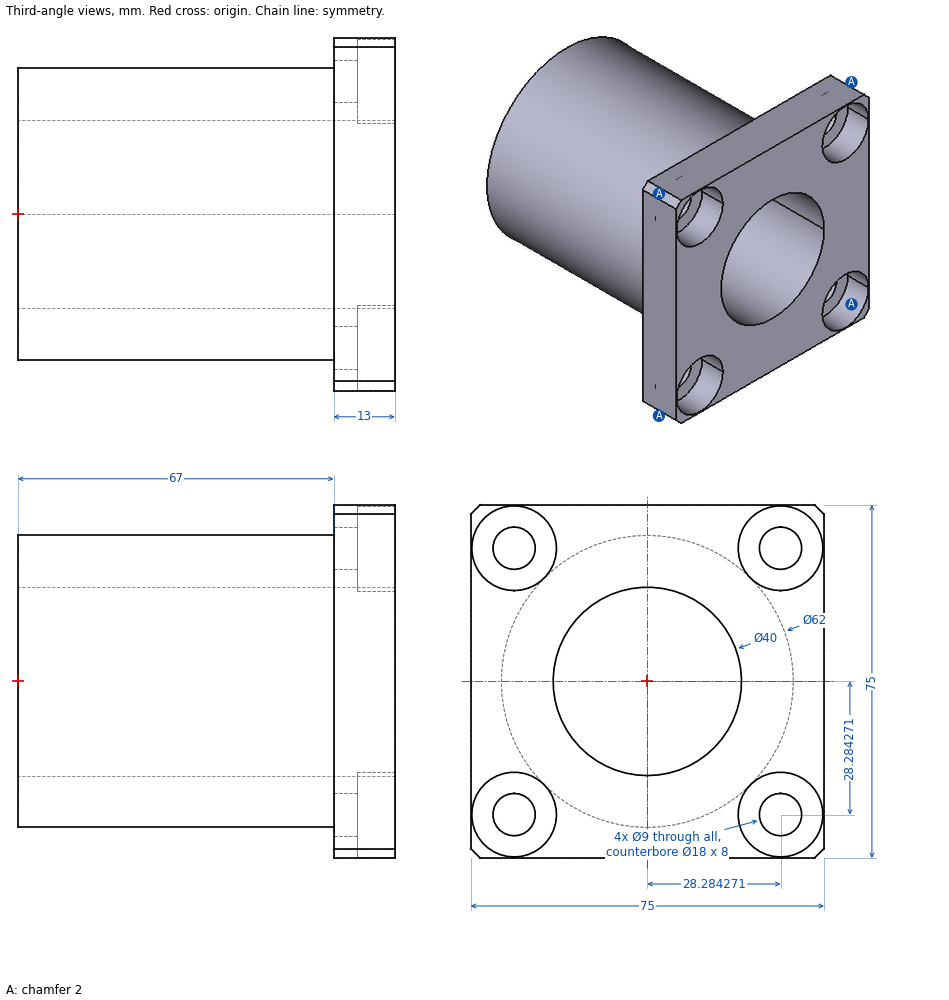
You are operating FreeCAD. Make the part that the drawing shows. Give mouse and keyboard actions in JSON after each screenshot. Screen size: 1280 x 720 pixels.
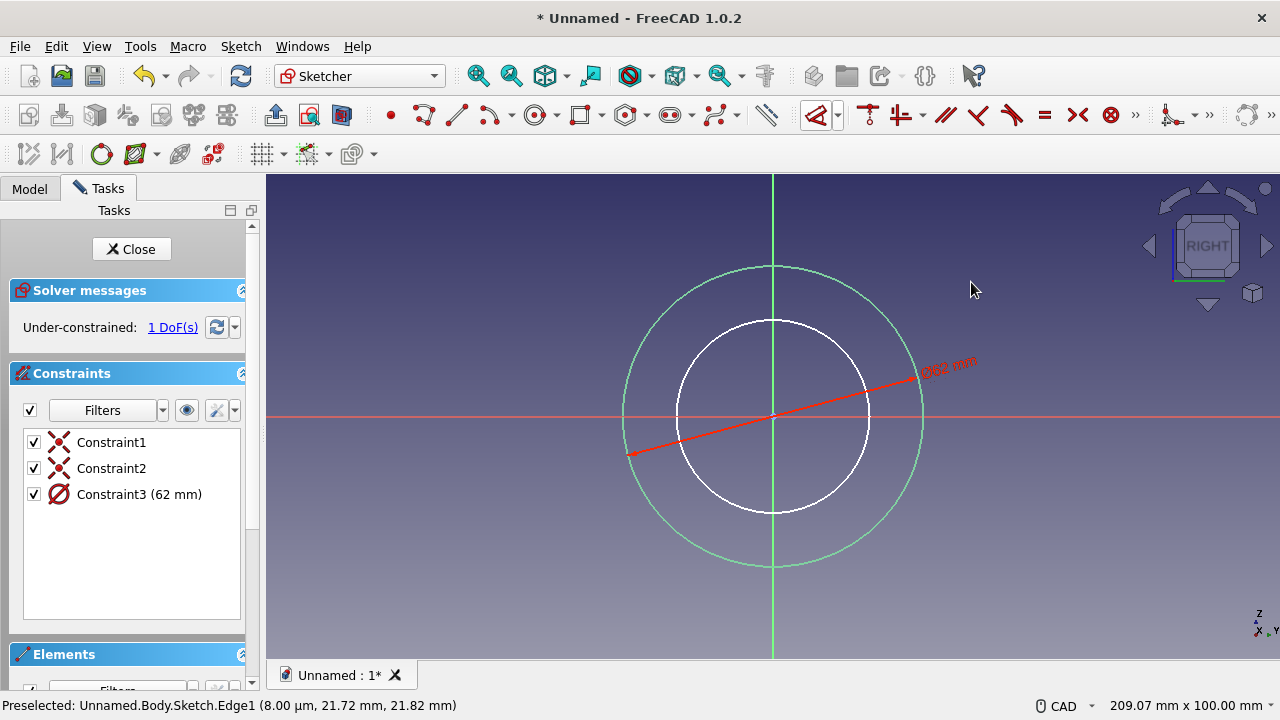
{"action": "left_click", "coordinate": [841, 348]}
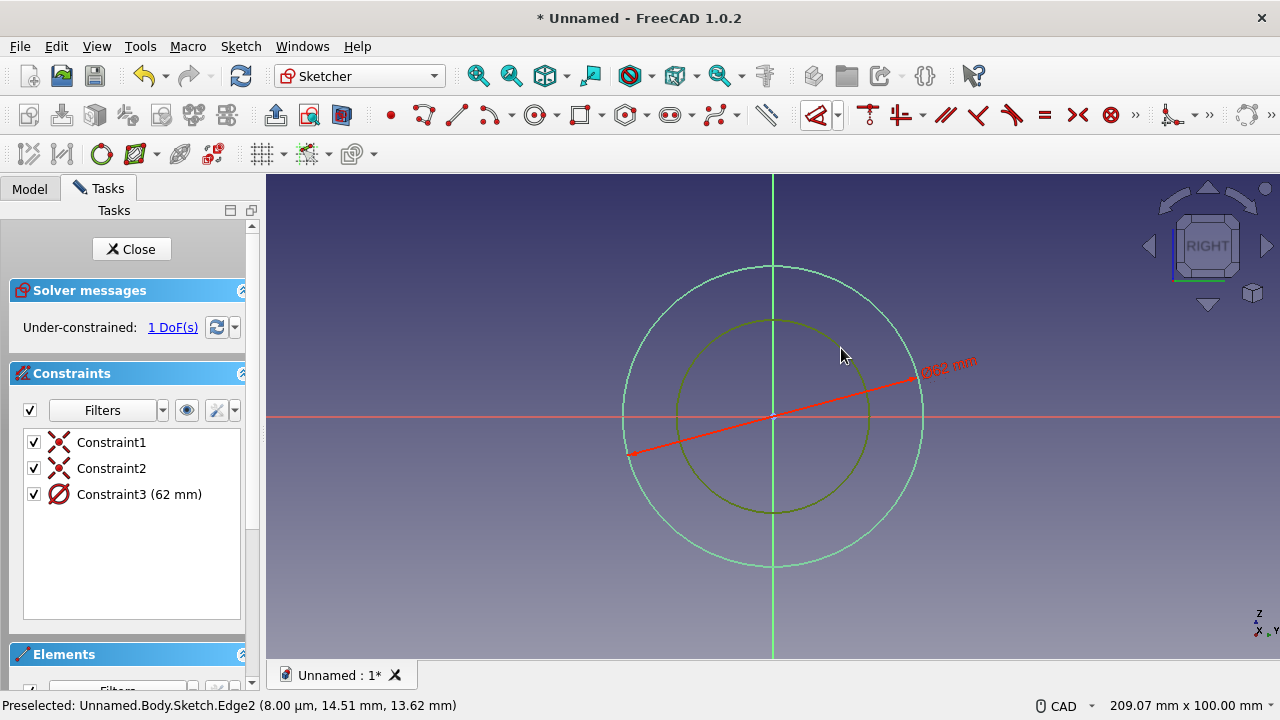
{"action": "key", "text": "k o"}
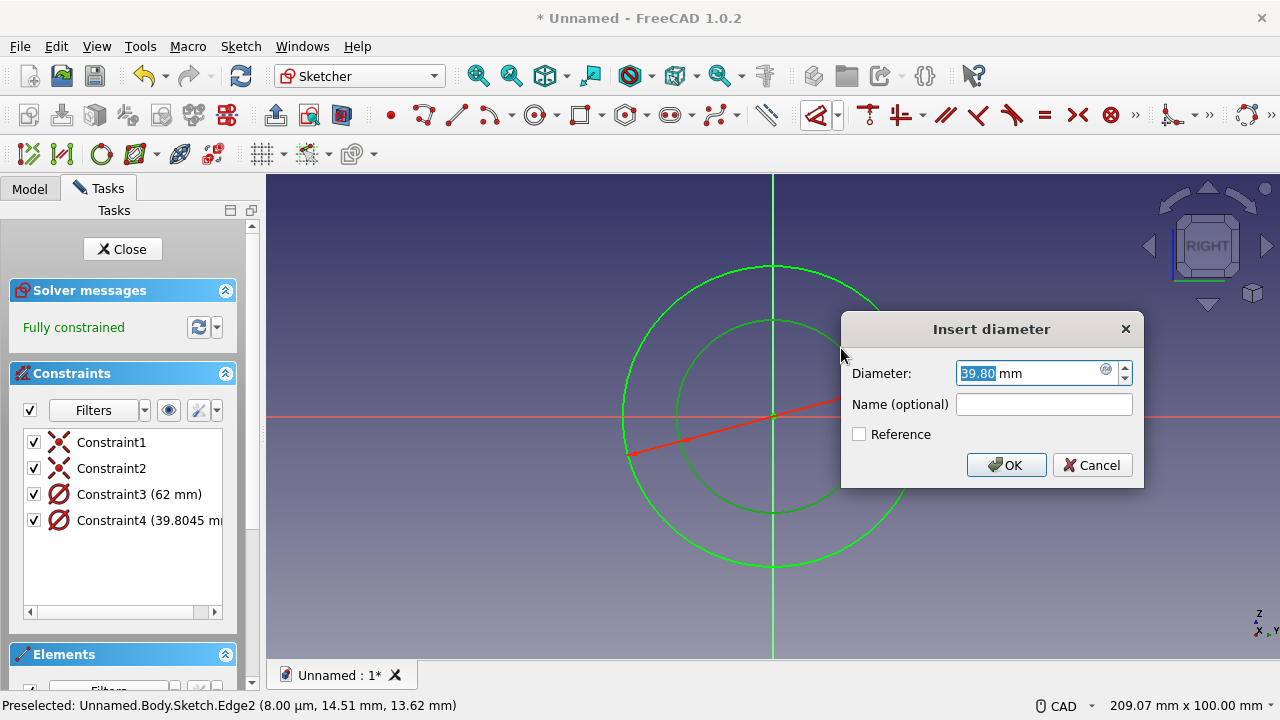
{"action": "type", "text": "40"}
{"action": "key", "text": "Return"}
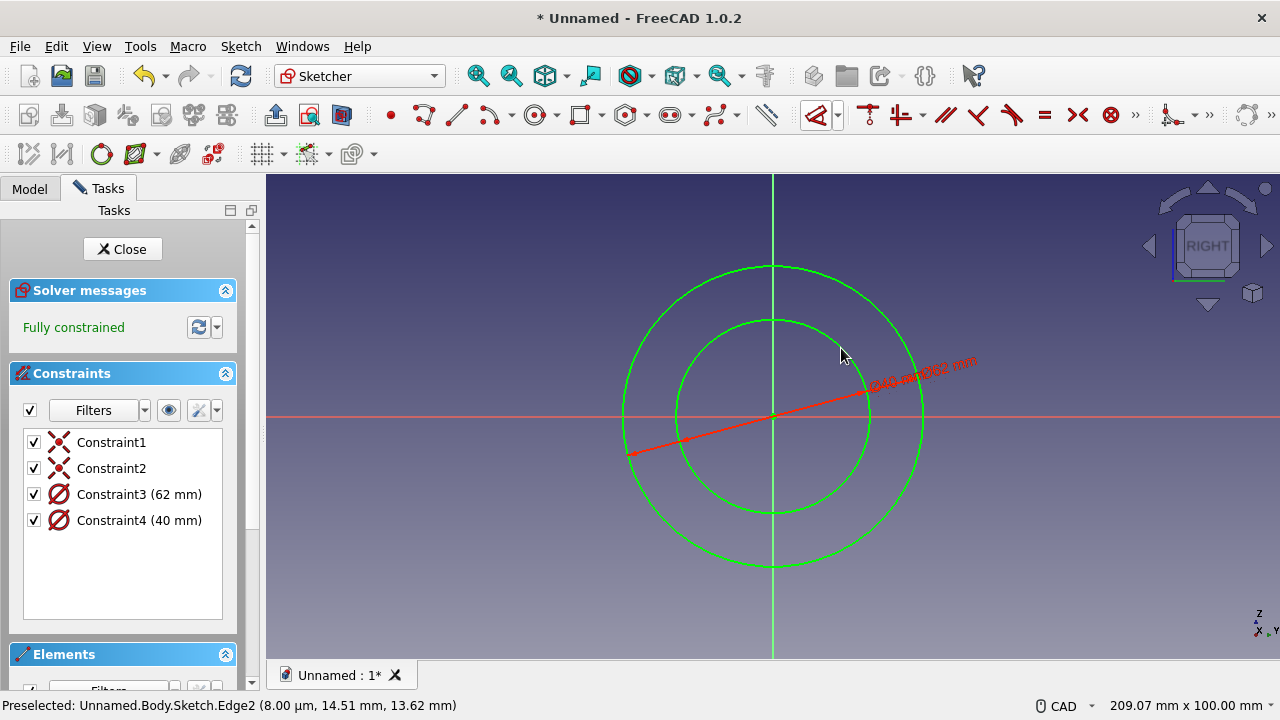
{"action": "left_click", "coordinate": [123, 249]}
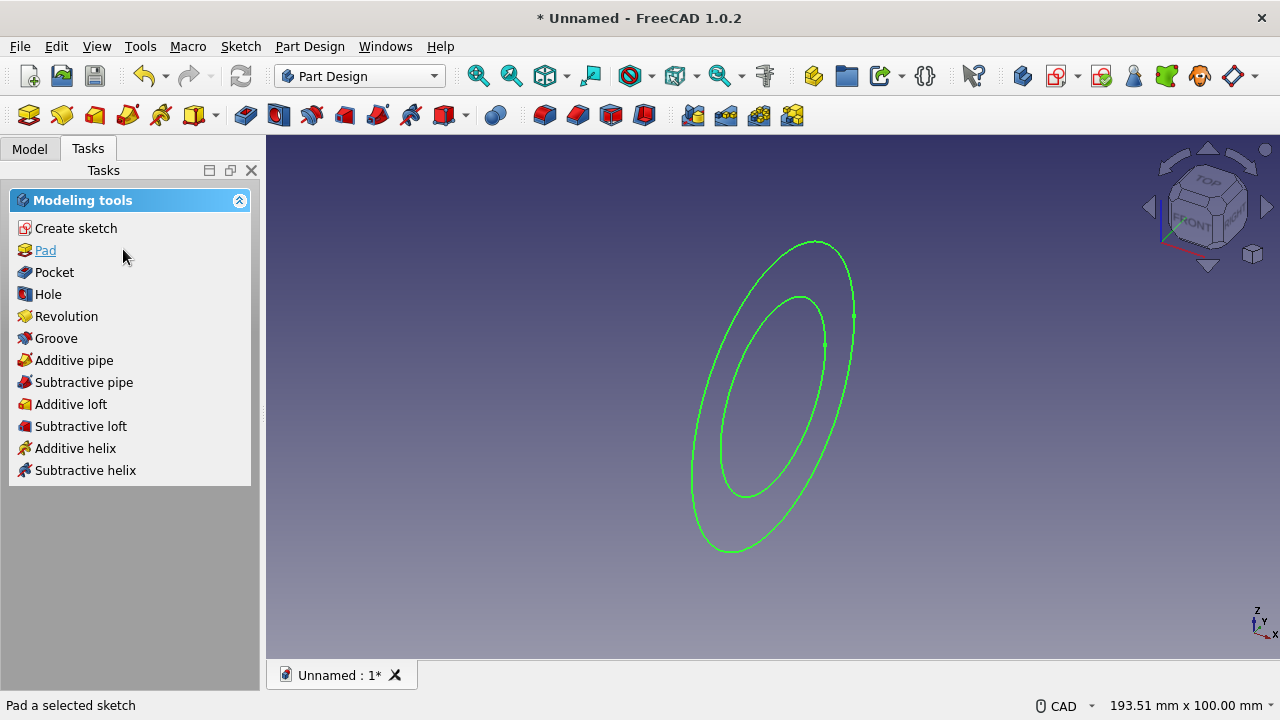
{"action": "left_click", "coordinate": [29, 116]}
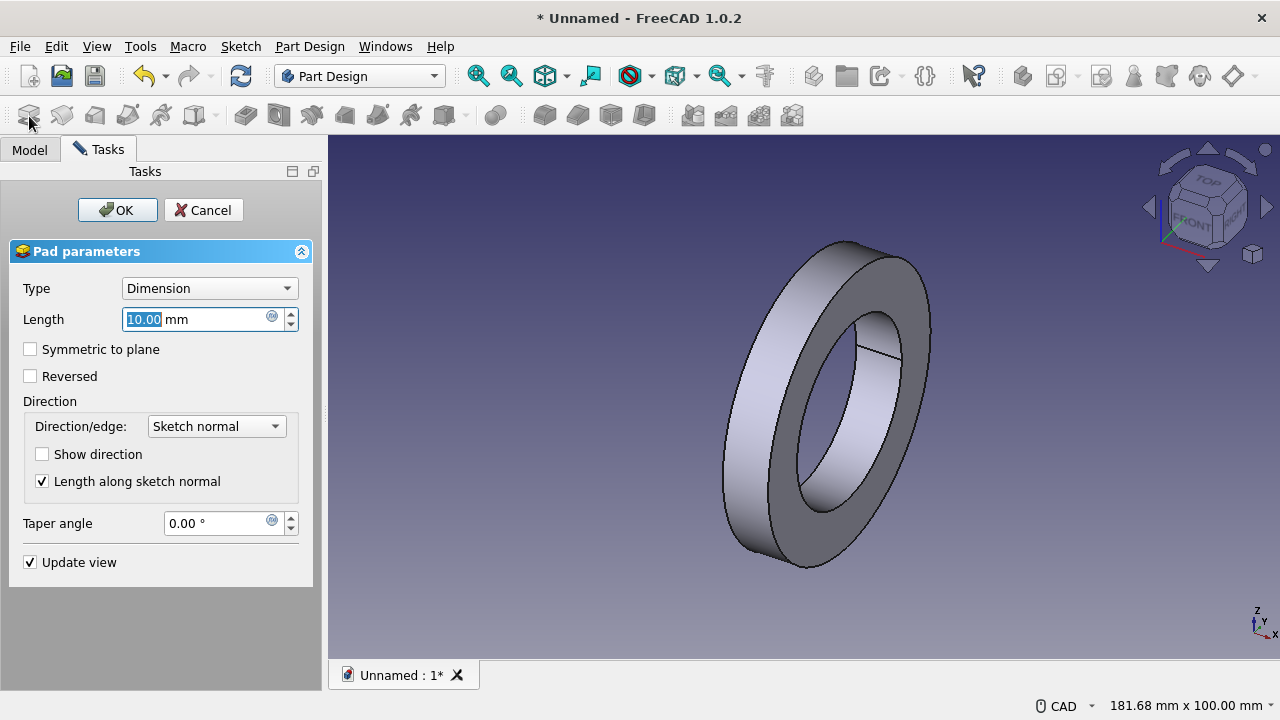
{"action": "type", "text": "67"}
{"action": "key", "text": "Tab"}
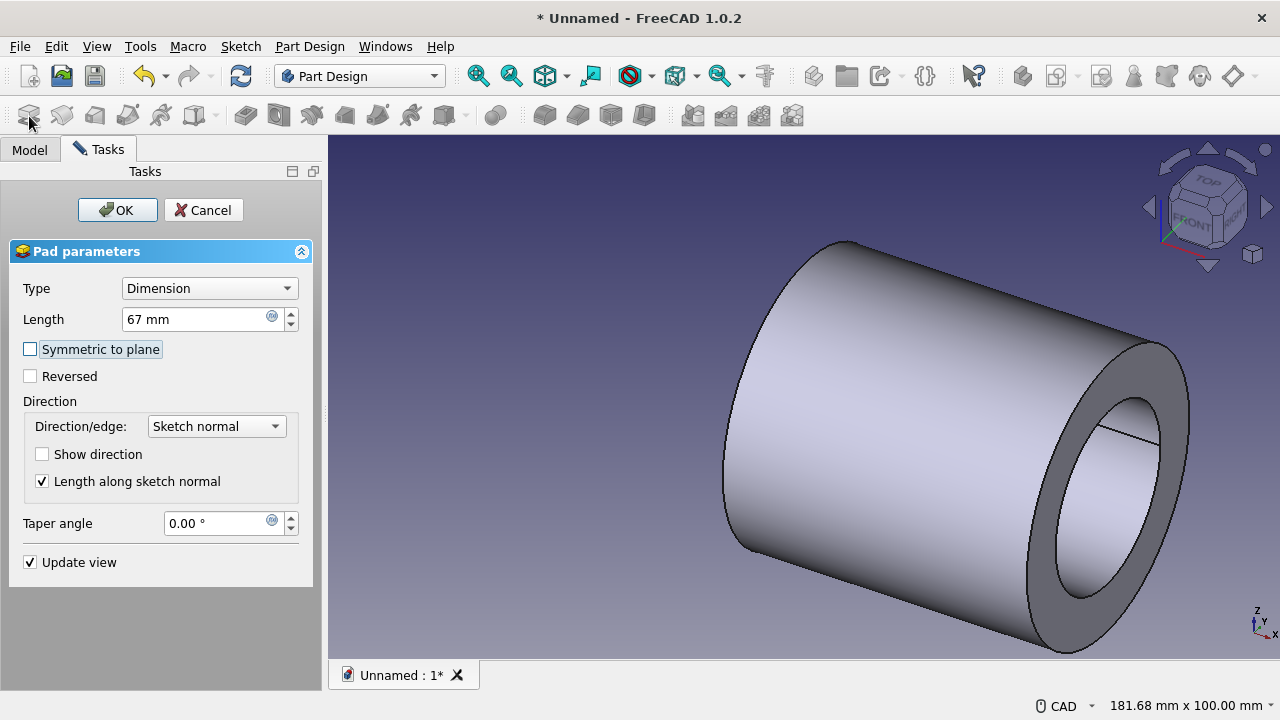
{"action": "left_click", "coordinate": [118, 210]}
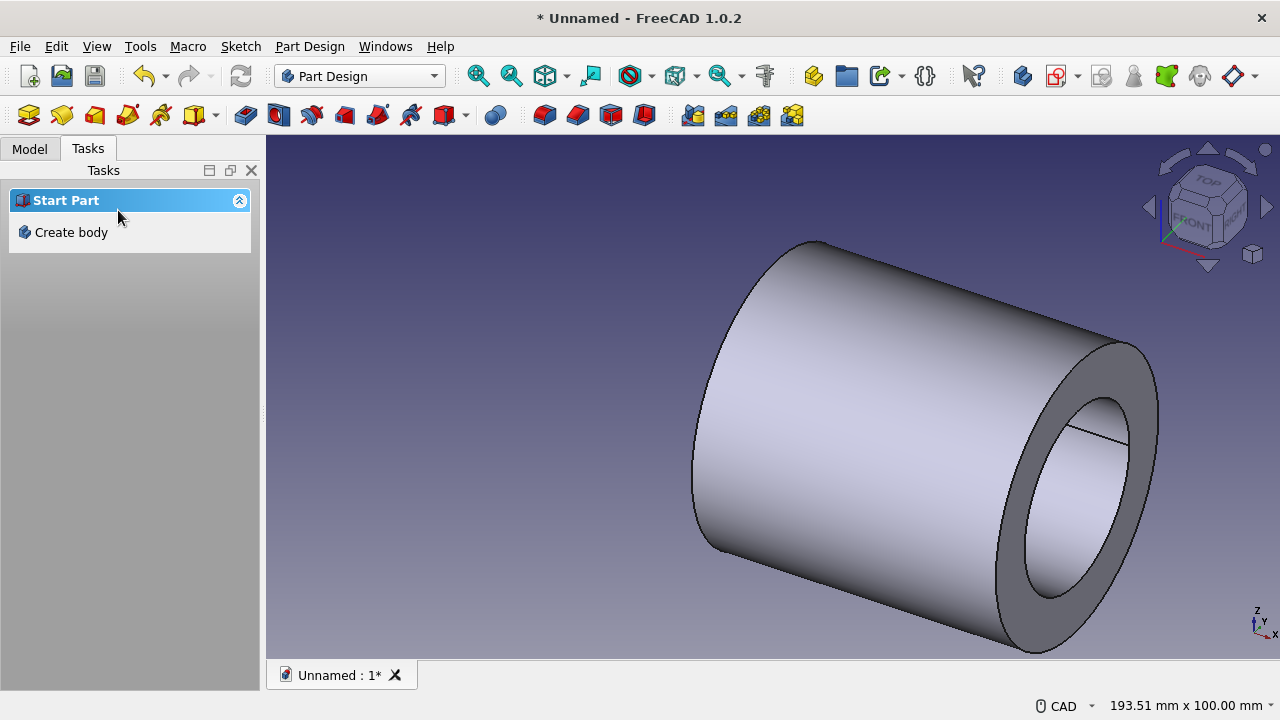
{"action": "left_click", "coordinate": [479, 76]}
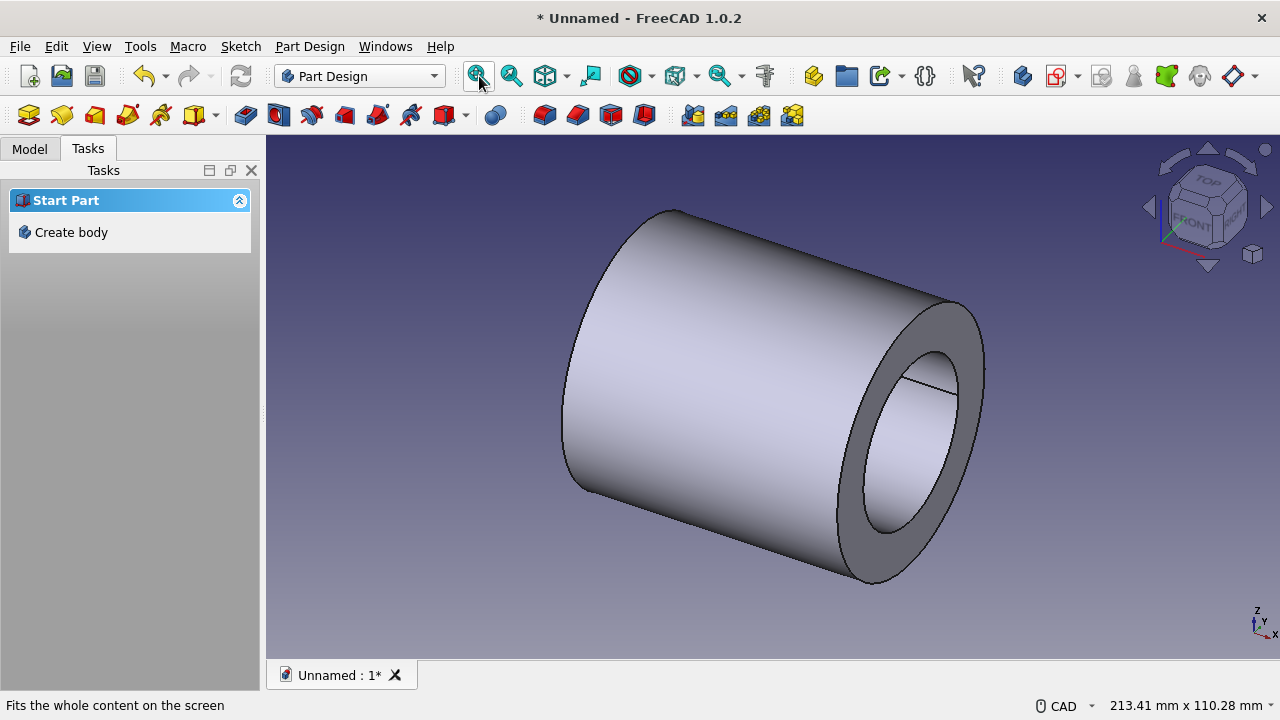
{"action": "left_click", "coordinate": [953, 331]}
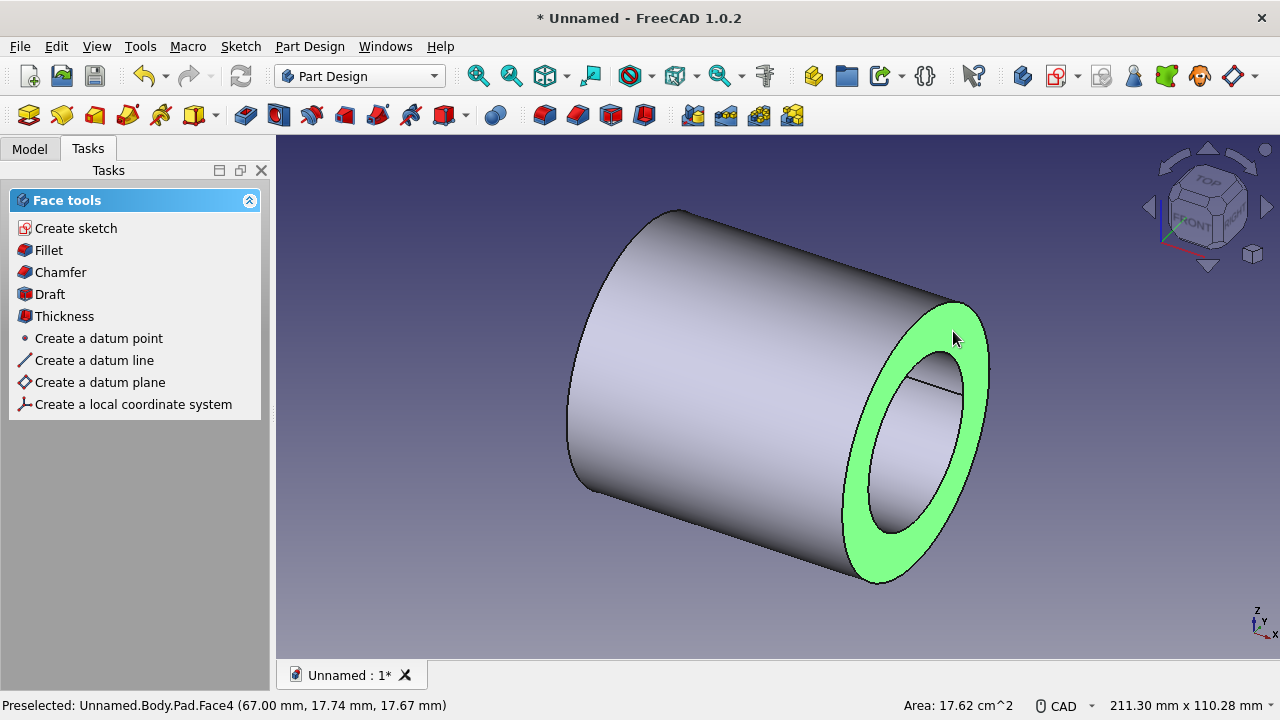
{"action": "left_click", "coordinate": [1056, 76]}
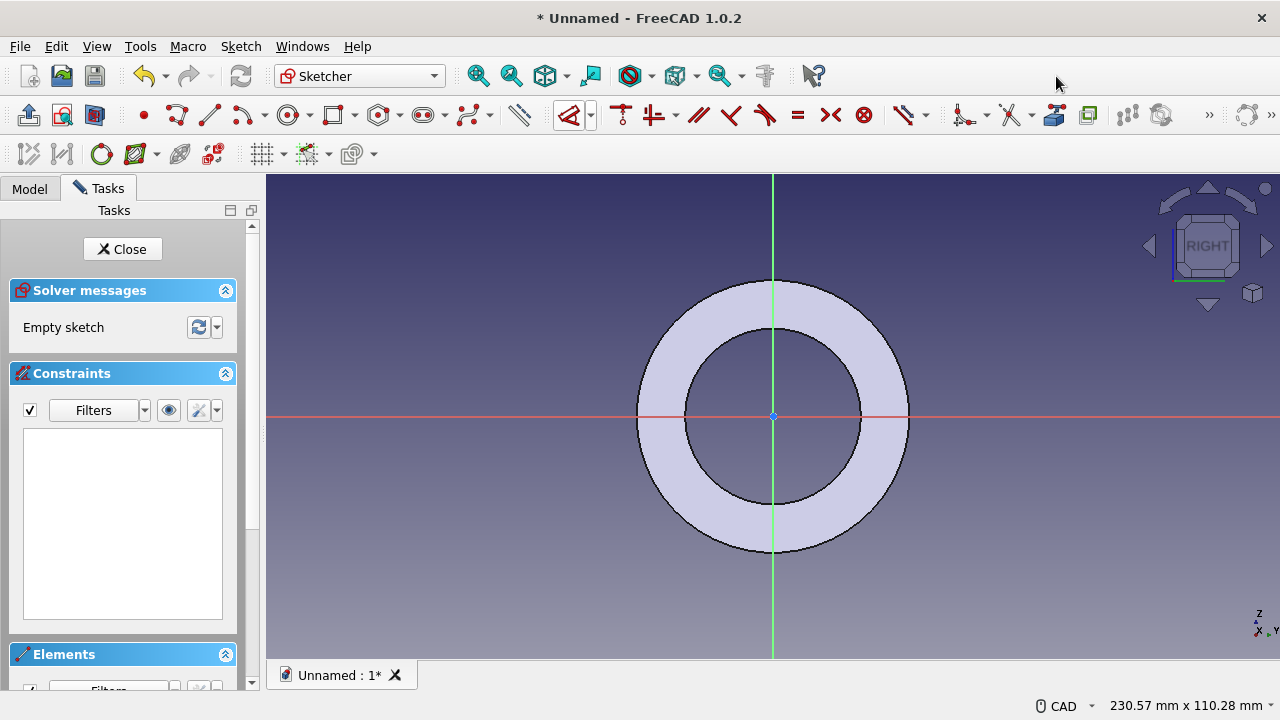
{"action": "left_click", "coordinate": [354, 116]}